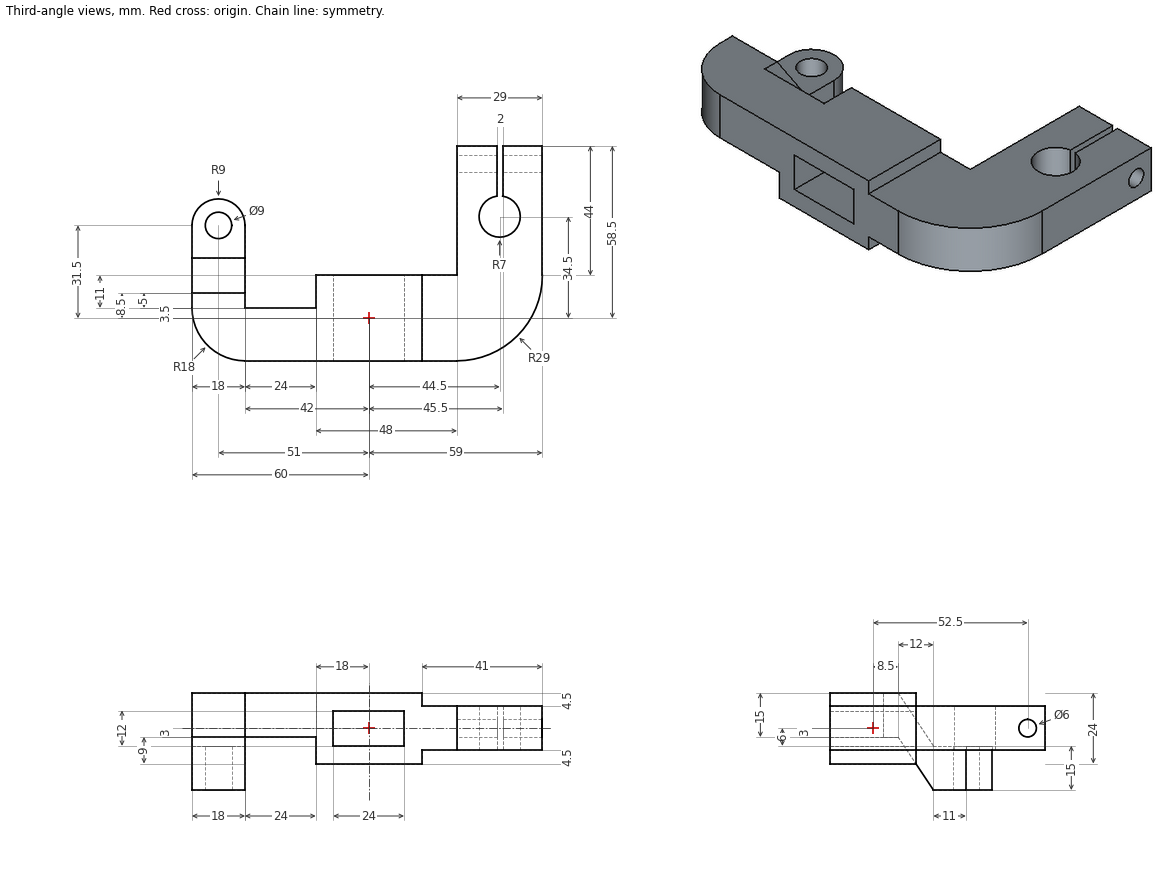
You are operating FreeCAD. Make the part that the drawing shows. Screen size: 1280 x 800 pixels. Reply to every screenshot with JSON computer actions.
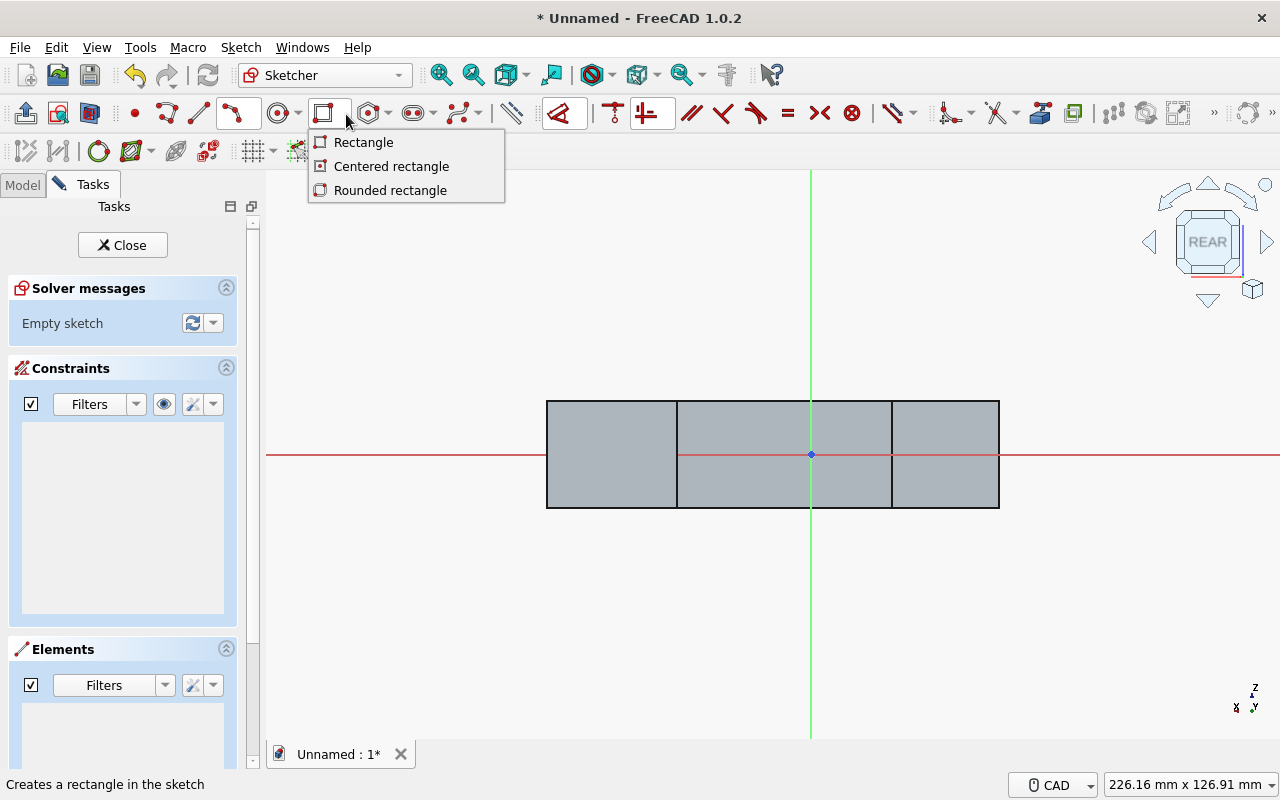
{"action": "left_click", "coordinate": [406, 166]}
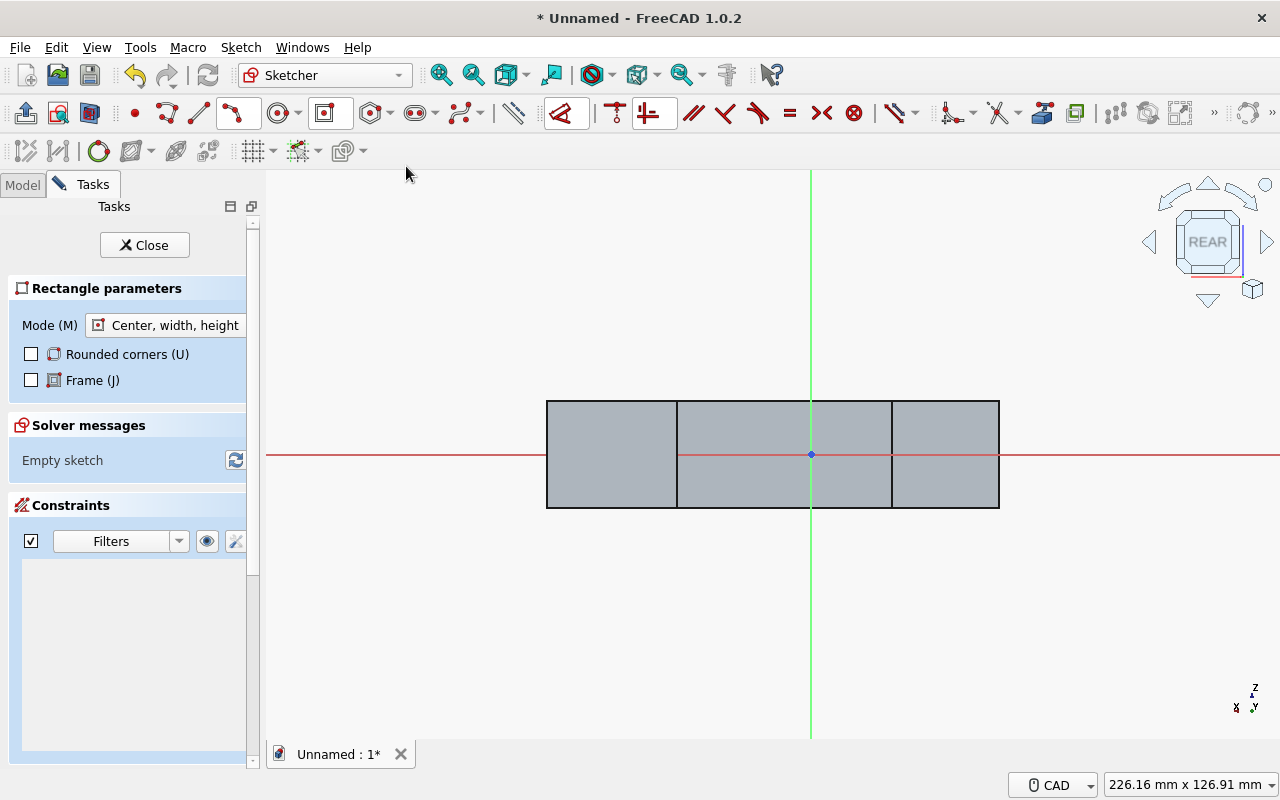
{"action": "left_click", "coordinate": [811, 454]}
{"action": "mouse_move", "coordinate": [865, 428]}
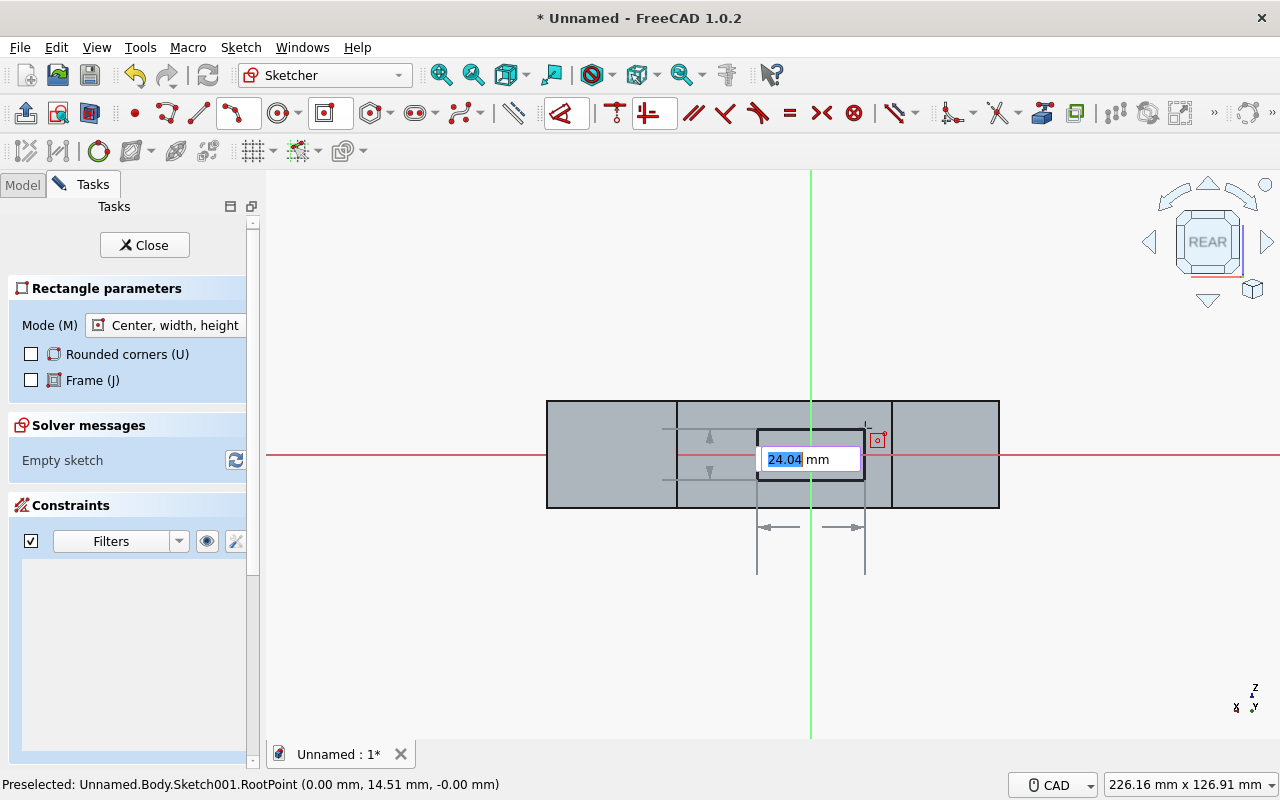
{"action": "type", "text": "24"}
{"action": "key", "text": "Tab"}
{"action": "type", "text": "12"}
{"action": "key", "text": "Return"}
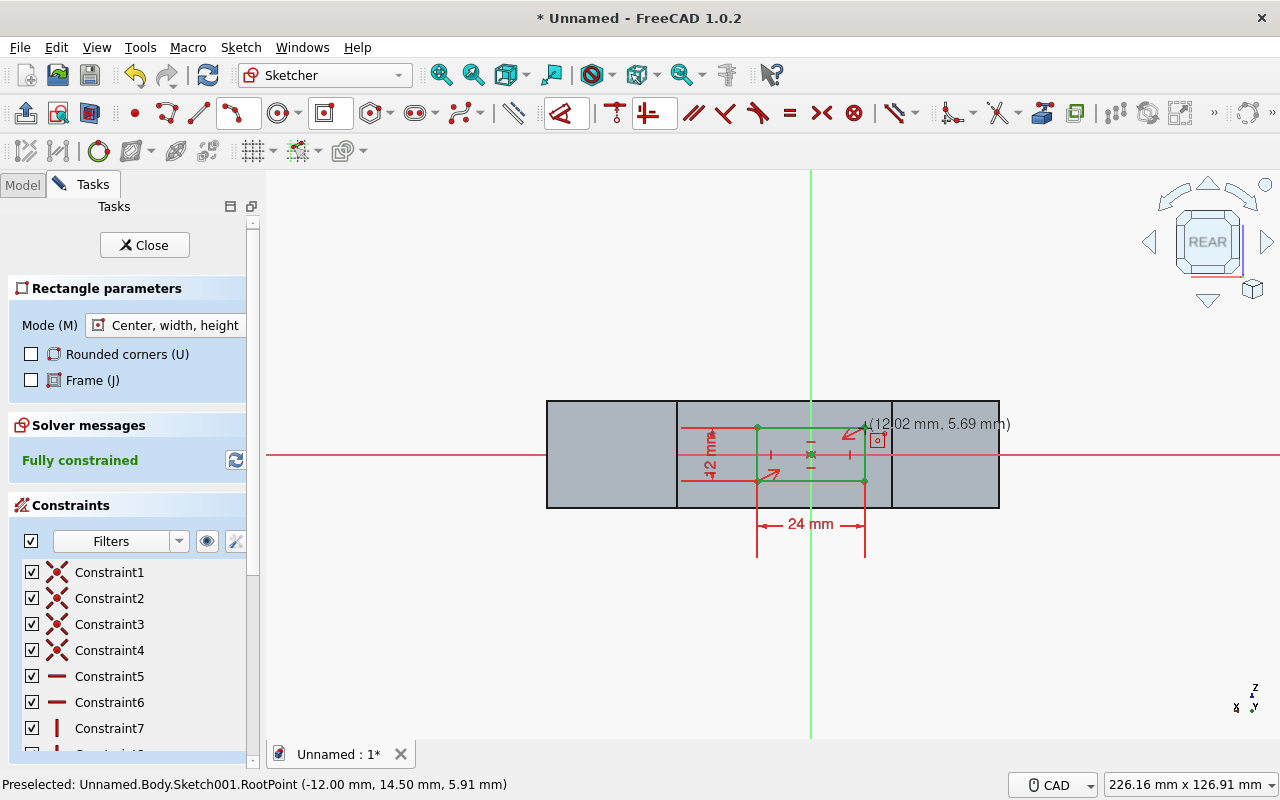
{"action": "left_click", "coordinate": [348, 114]}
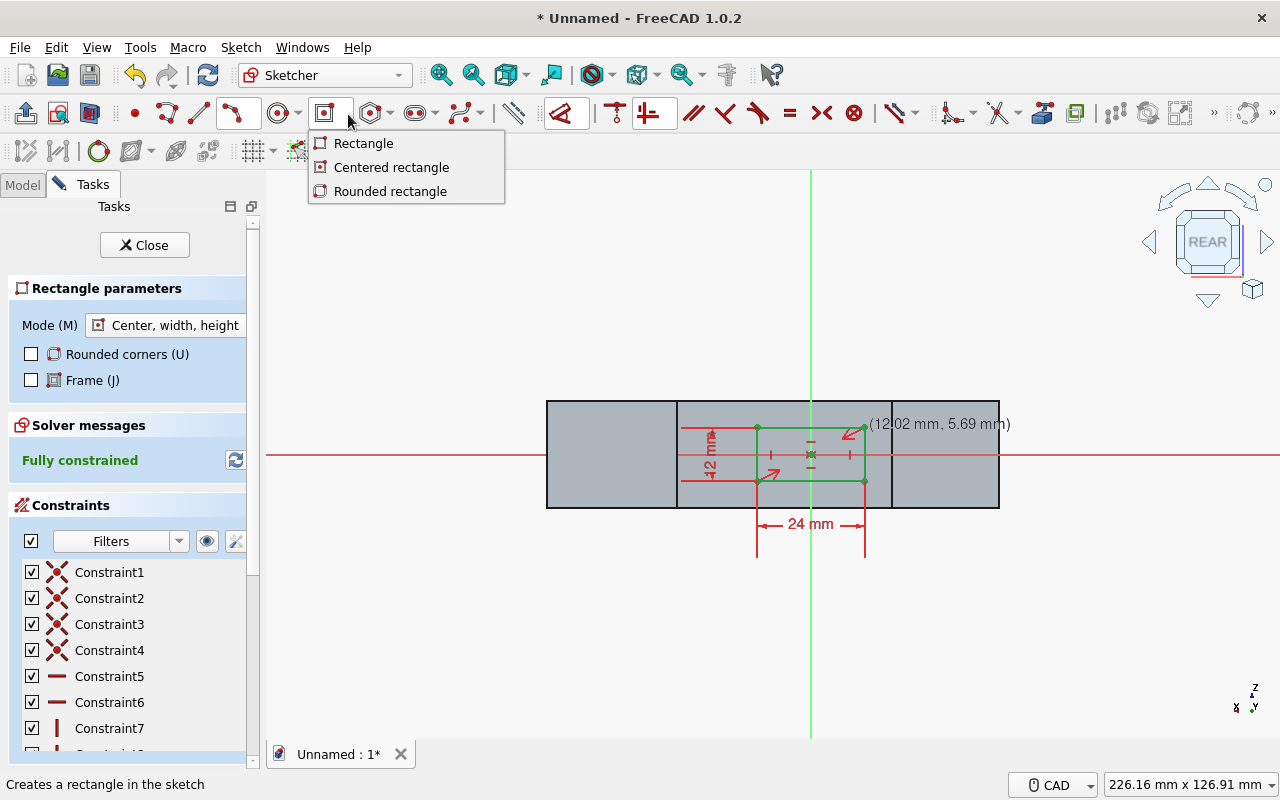
{"action": "left_click", "coordinate": [406, 143]}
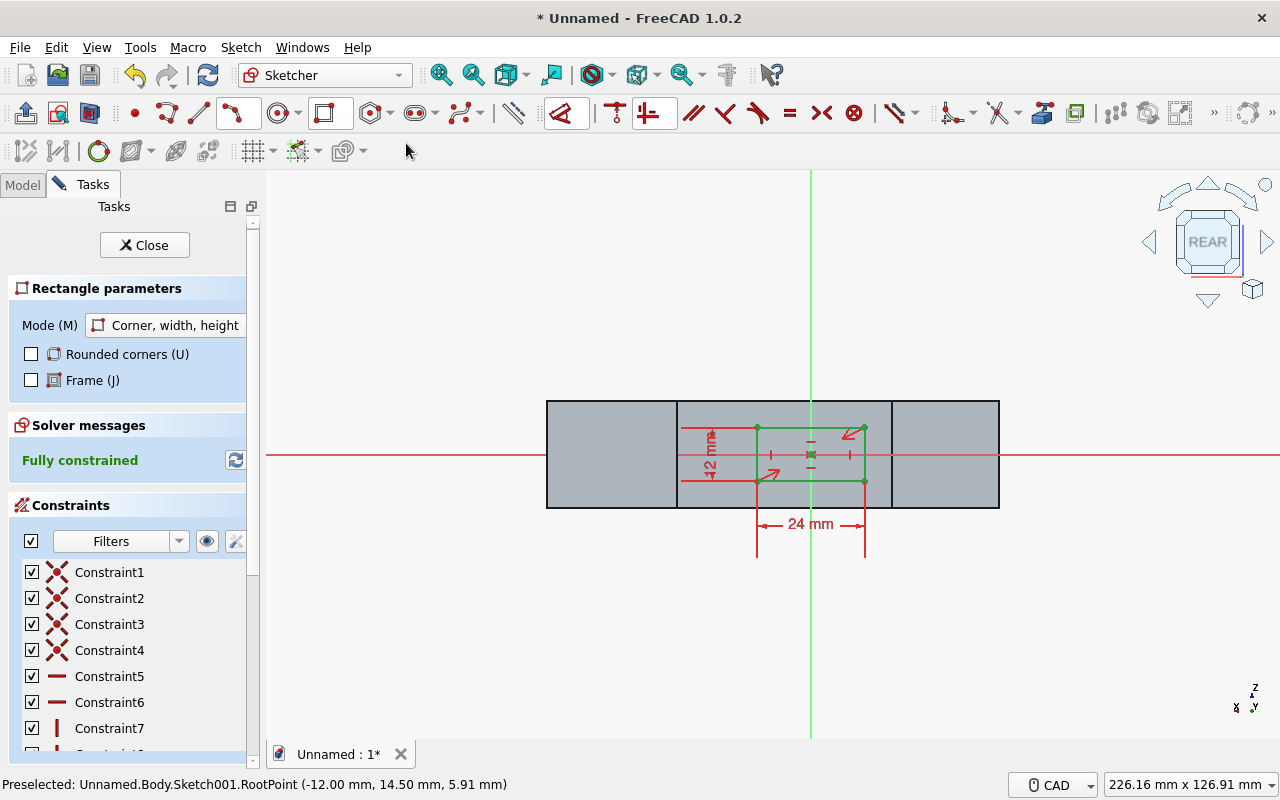
{"action": "left_click", "coordinate": [892, 468]}
{"action": "mouse_move", "coordinate": [999, 508]}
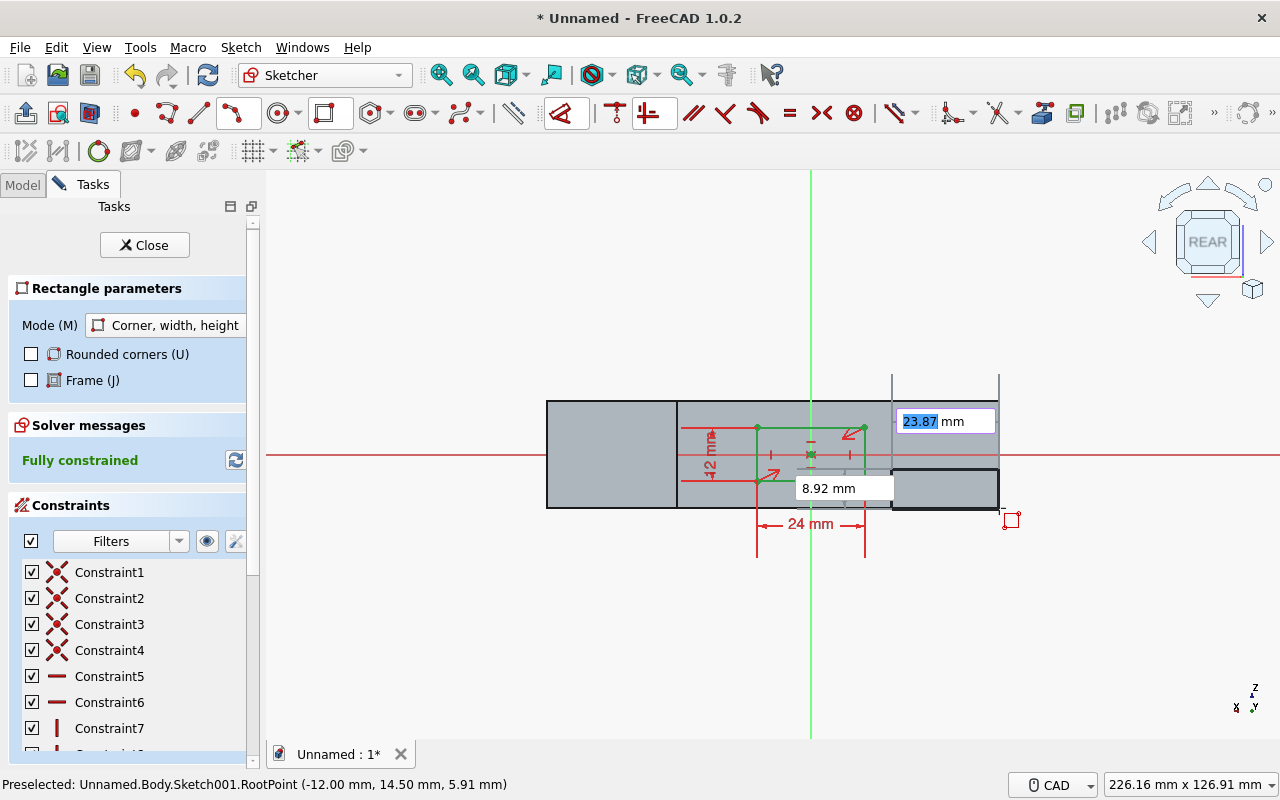
{"action": "type", "text": "24"}
{"action": "key", "text": "Tab"}
{"action": "type", "text": "9"}
{"action": "key", "text": "Return"}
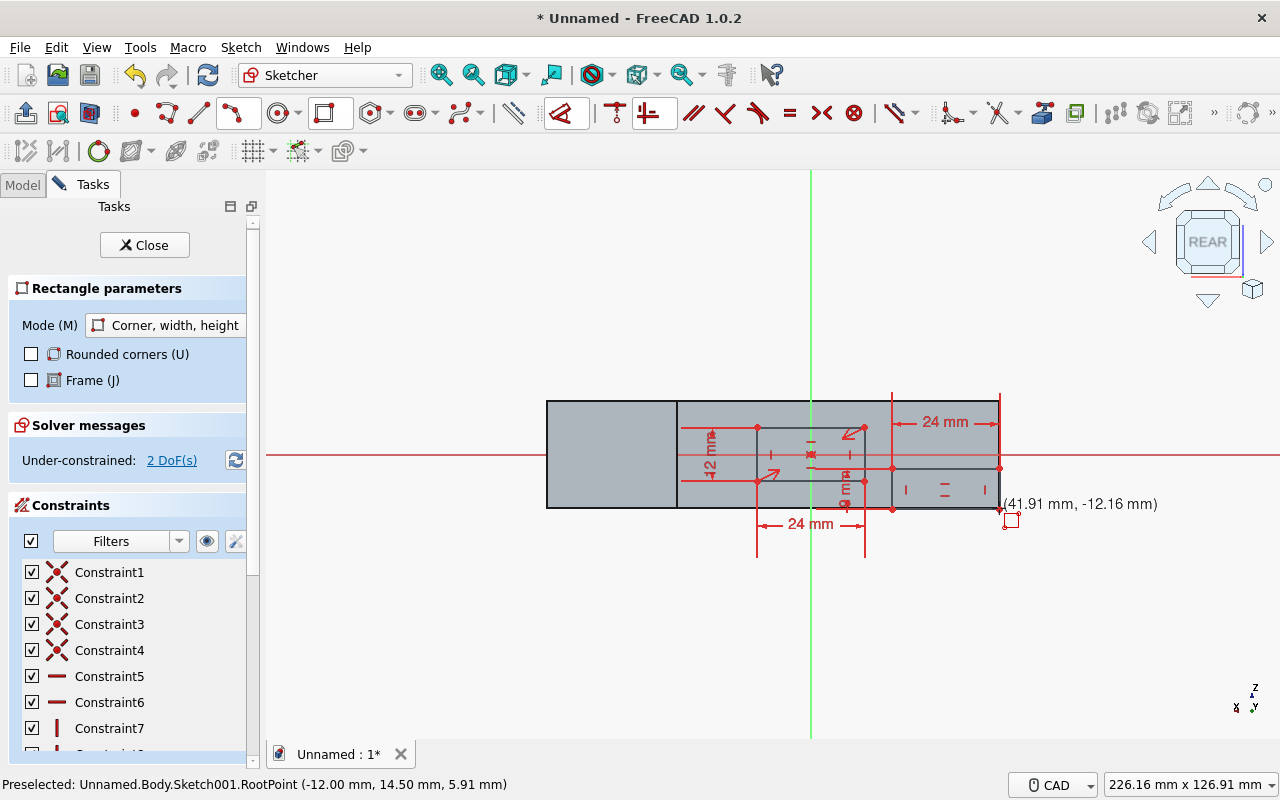
{"action": "left_click", "coordinate": [547, 401]}
{"action": "mouse_move", "coordinate": [730, 421]}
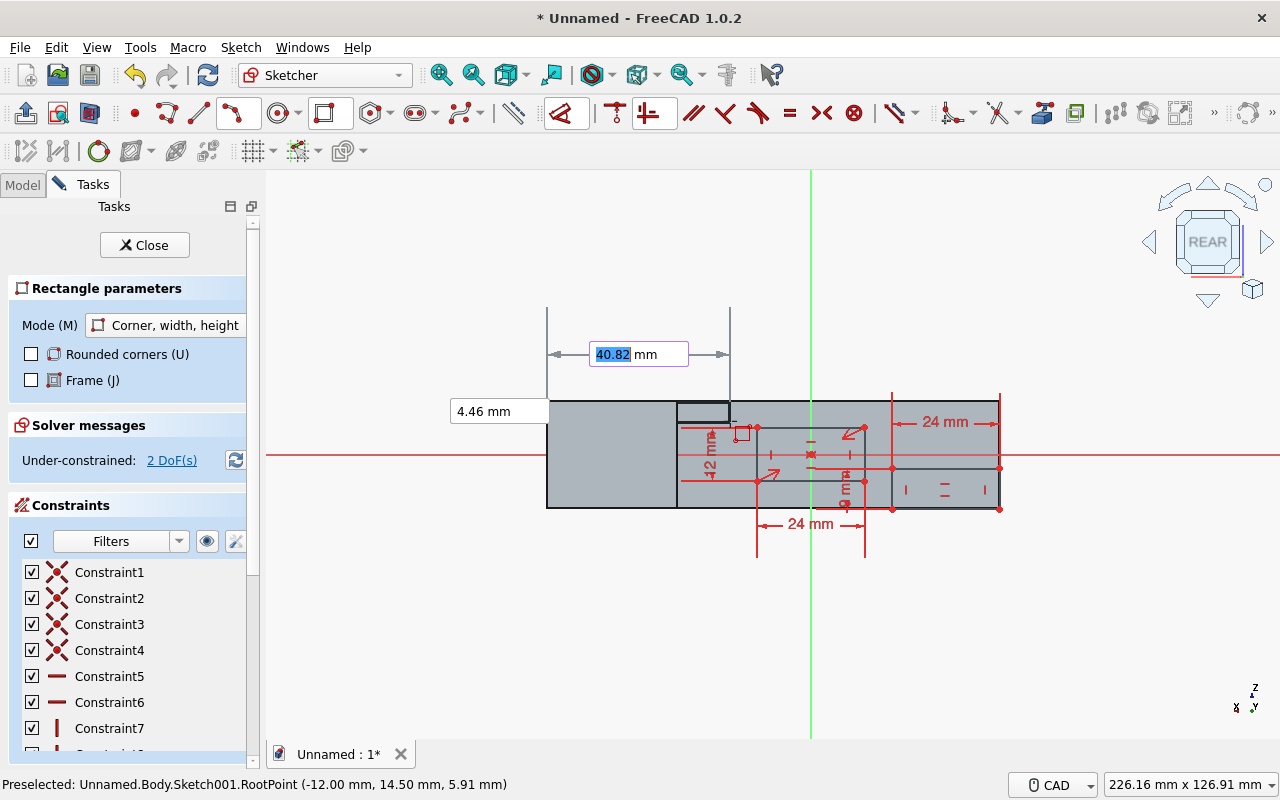
{"action": "type", "text": "41"}
{"action": "key", "text": "Tab"}
{"action": "type", "text": "4.5"}
{"action": "key", "text": "Return"}